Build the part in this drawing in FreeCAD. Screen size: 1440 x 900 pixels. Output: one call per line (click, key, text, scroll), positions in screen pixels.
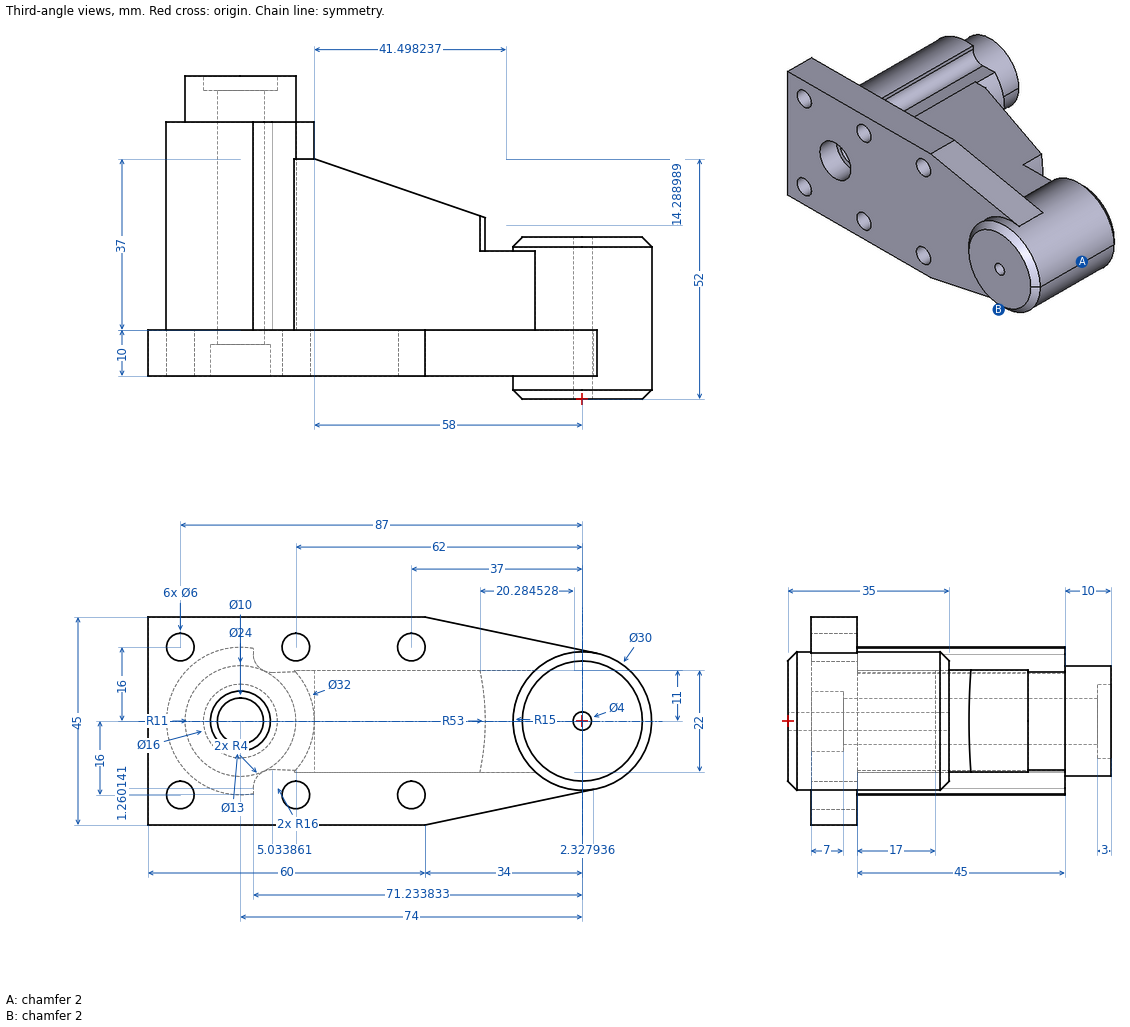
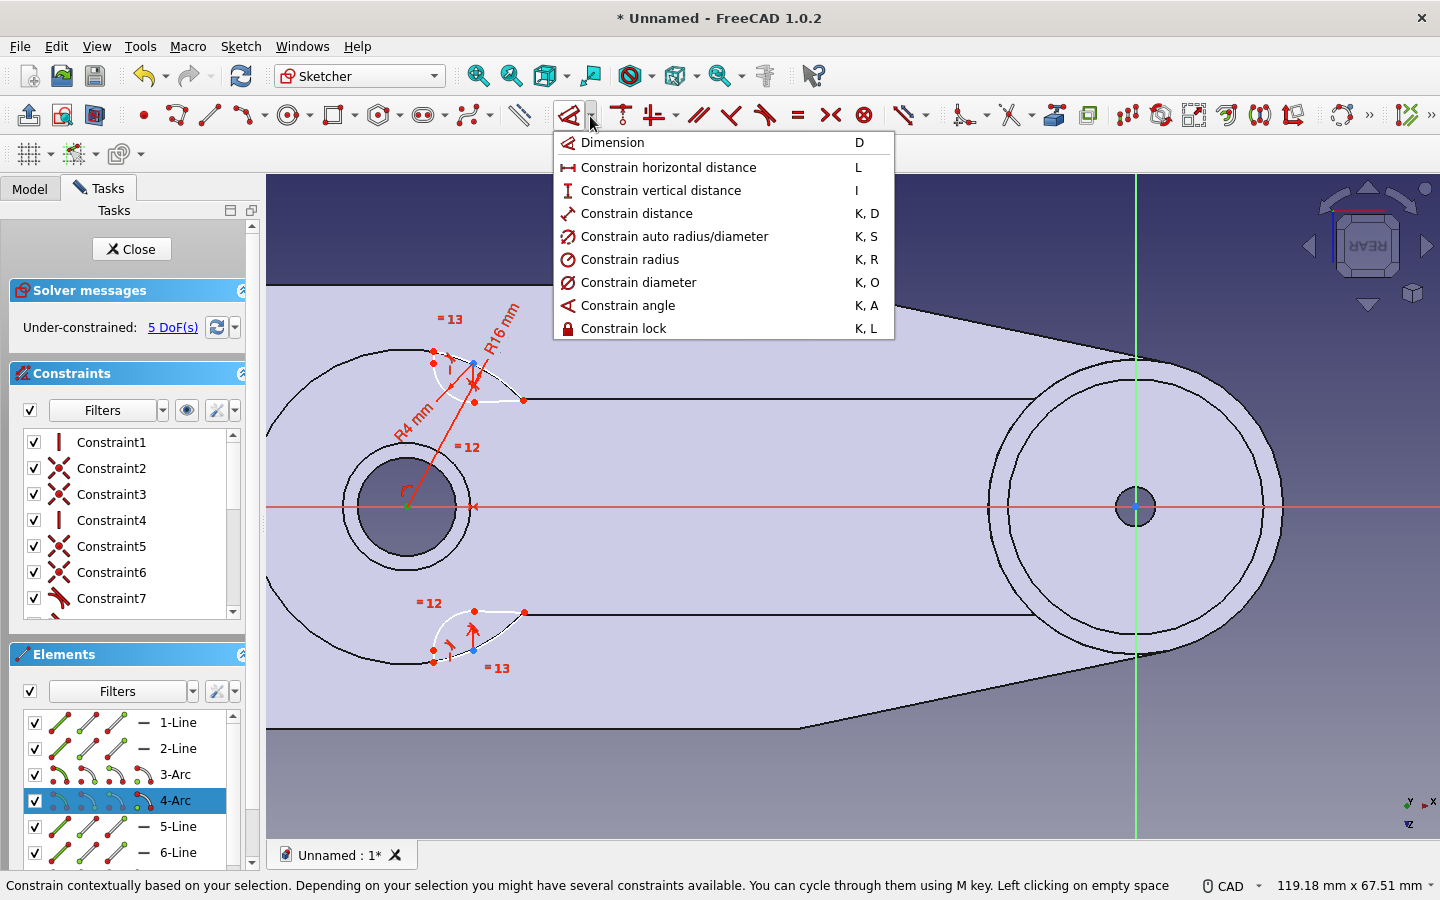
click(724, 168)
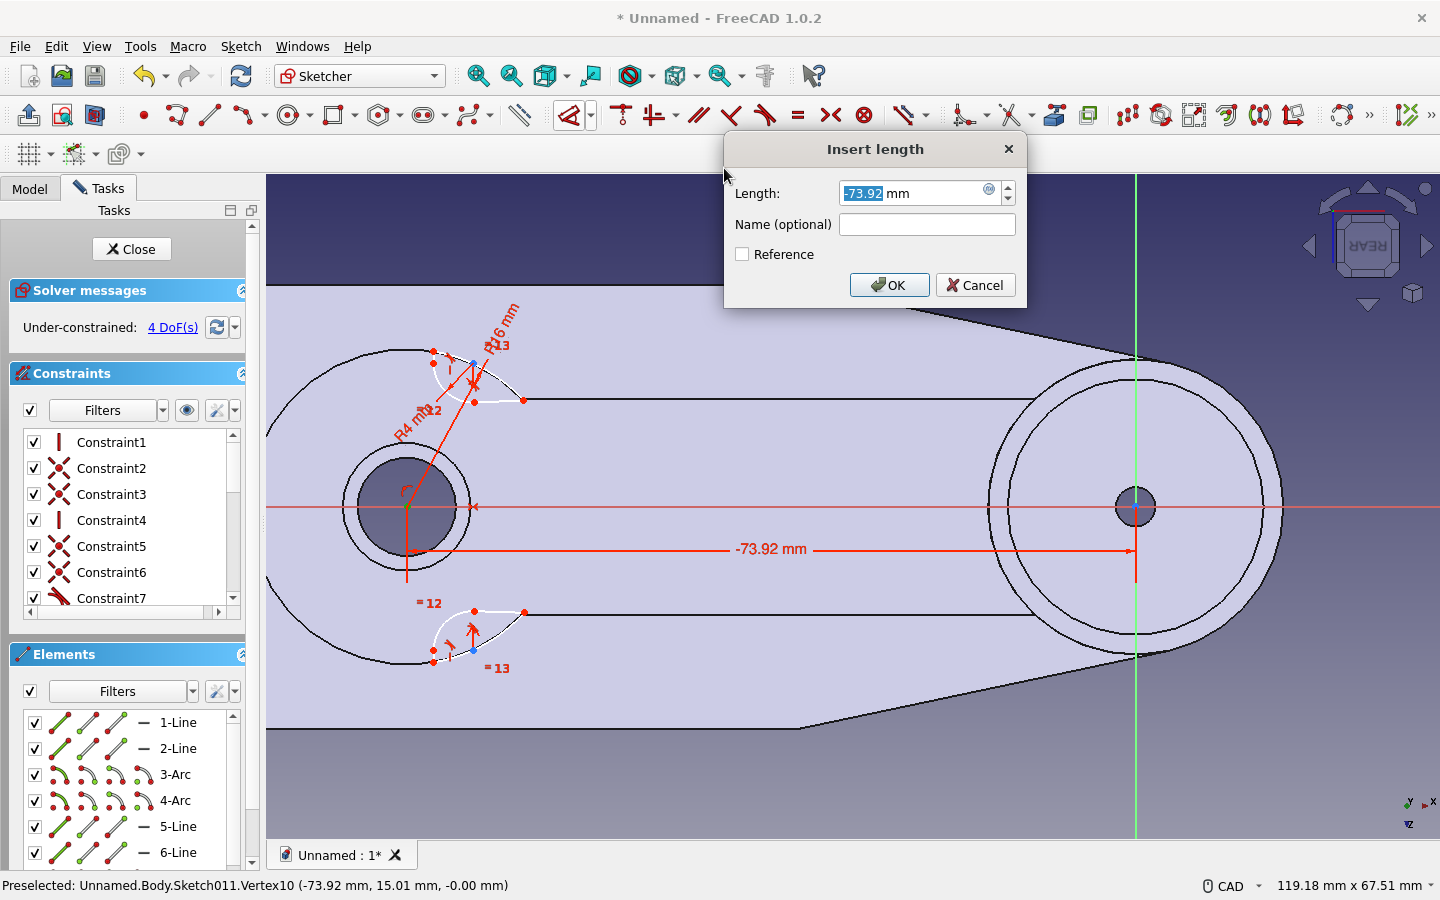
text(-74)
key(Return)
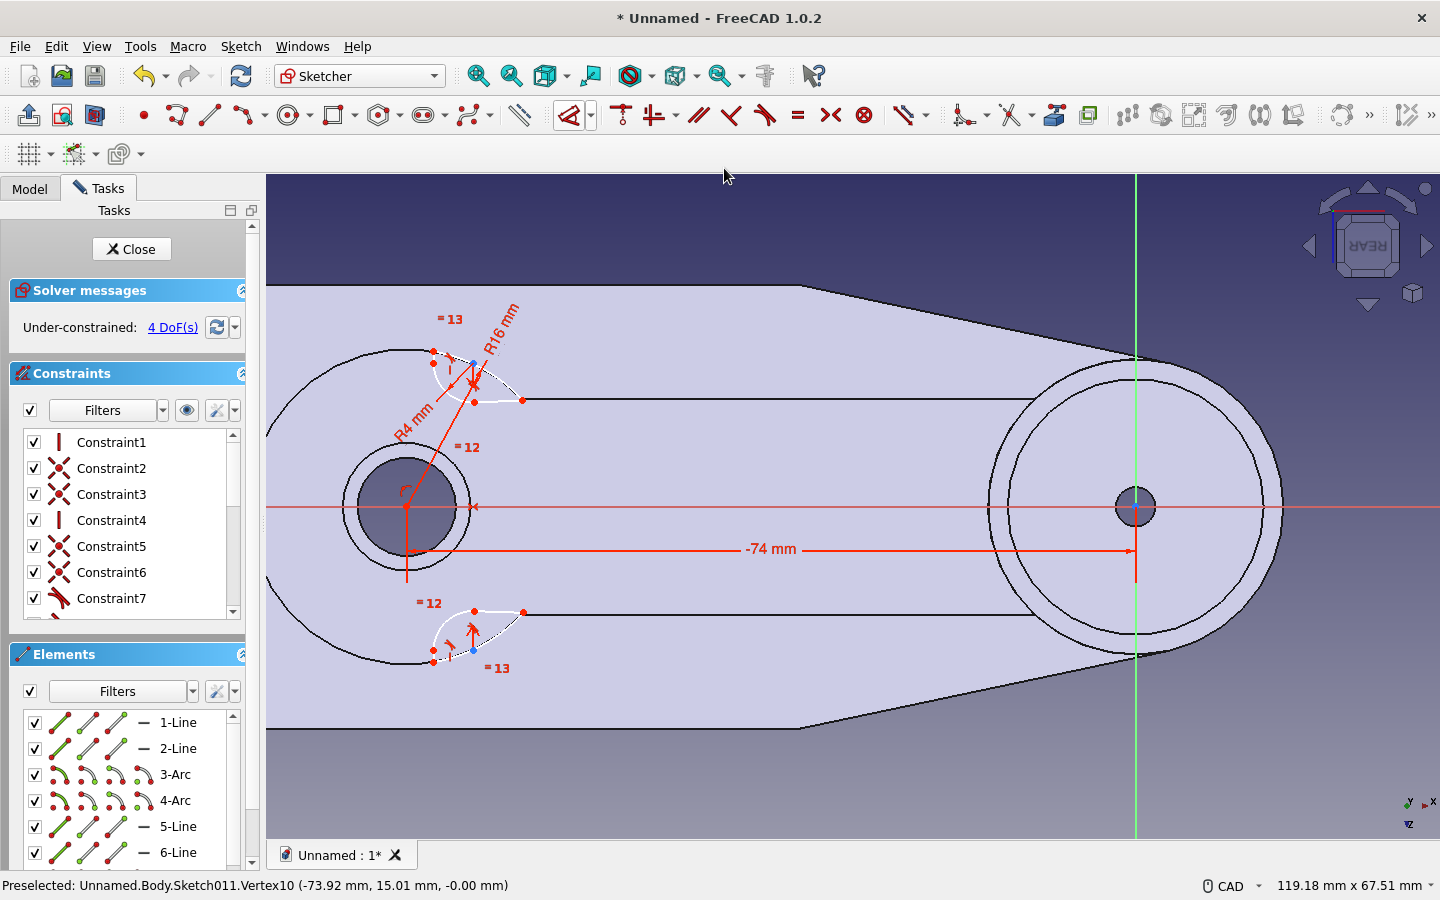
scroll(434, 357, up, 6)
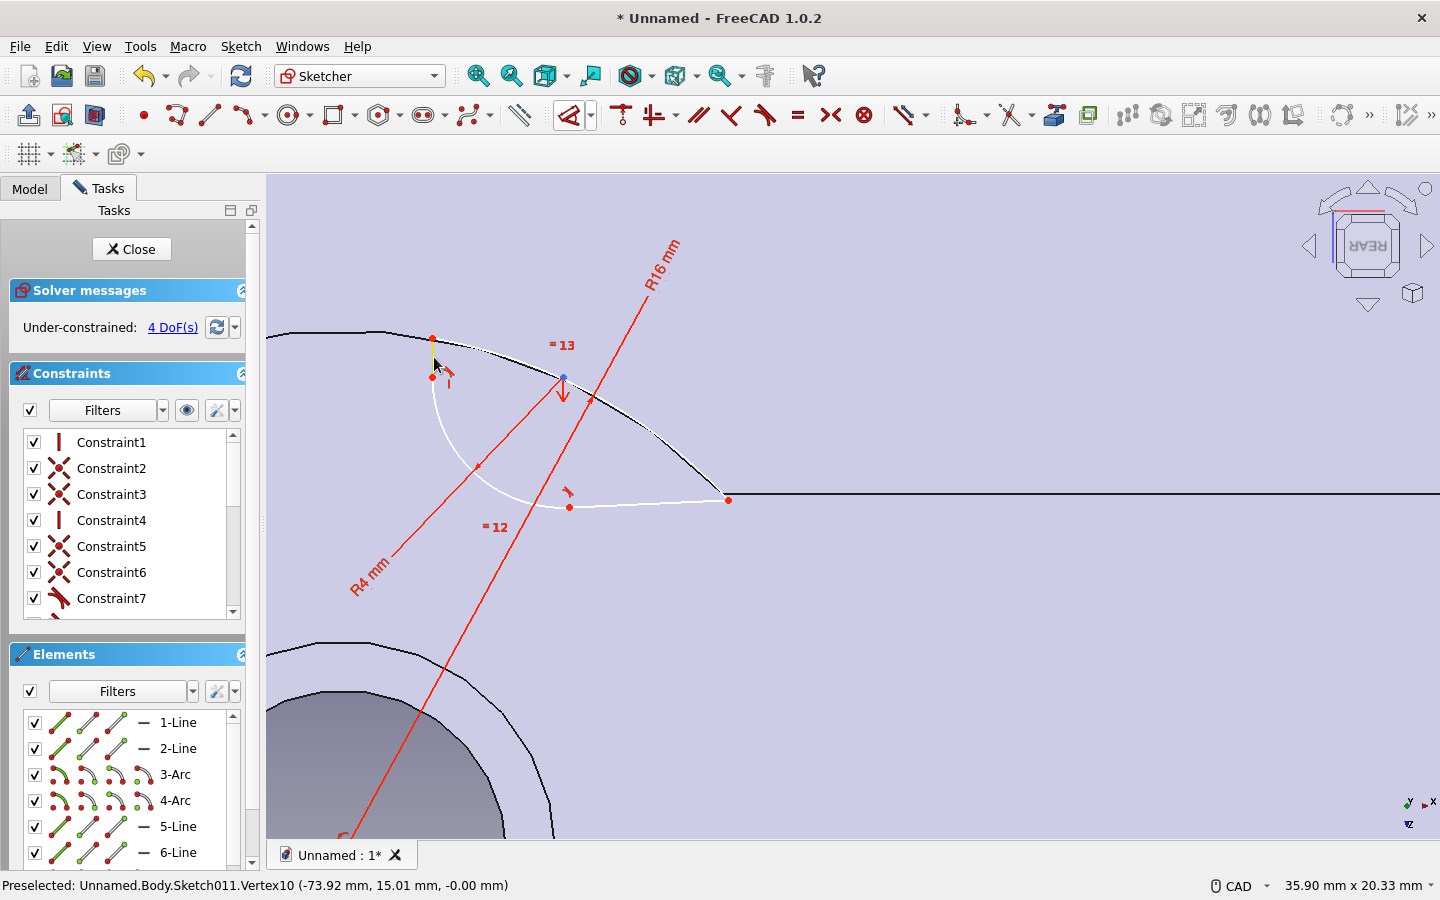
click(433, 358)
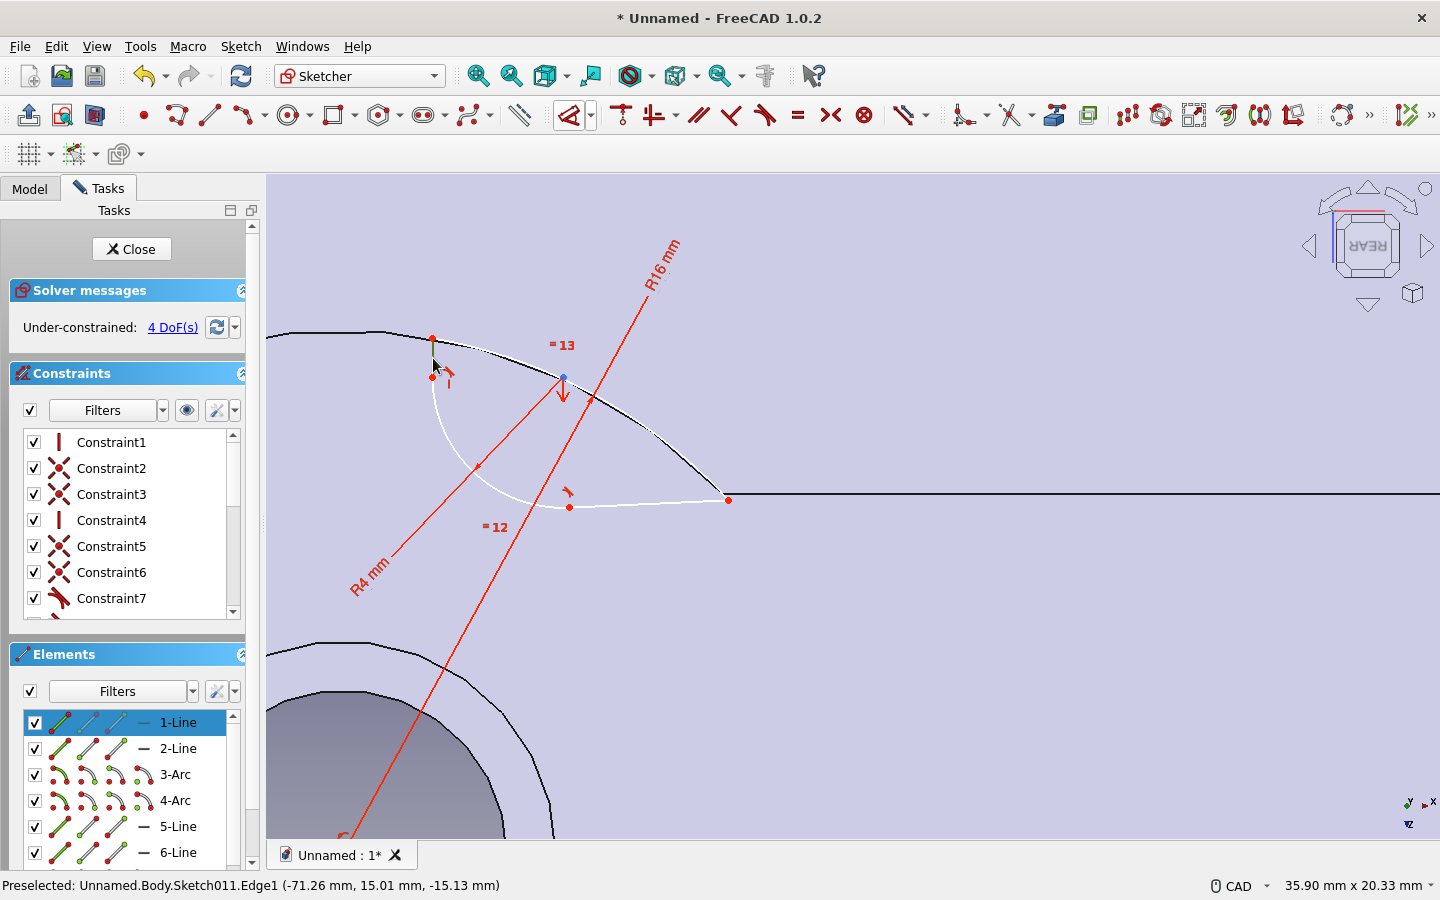
click(590, 116)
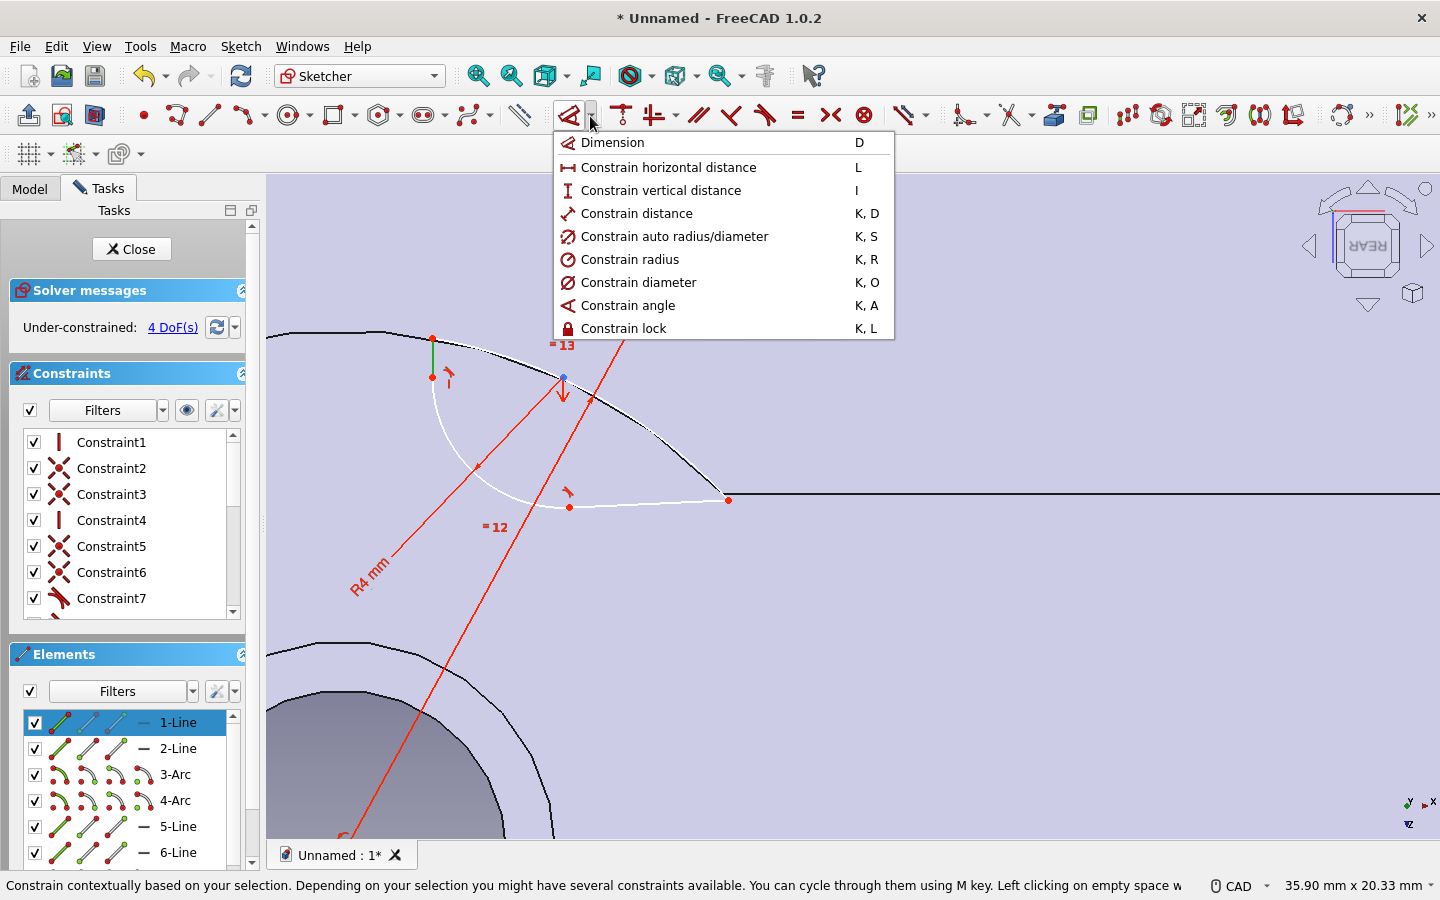
click(724, 190)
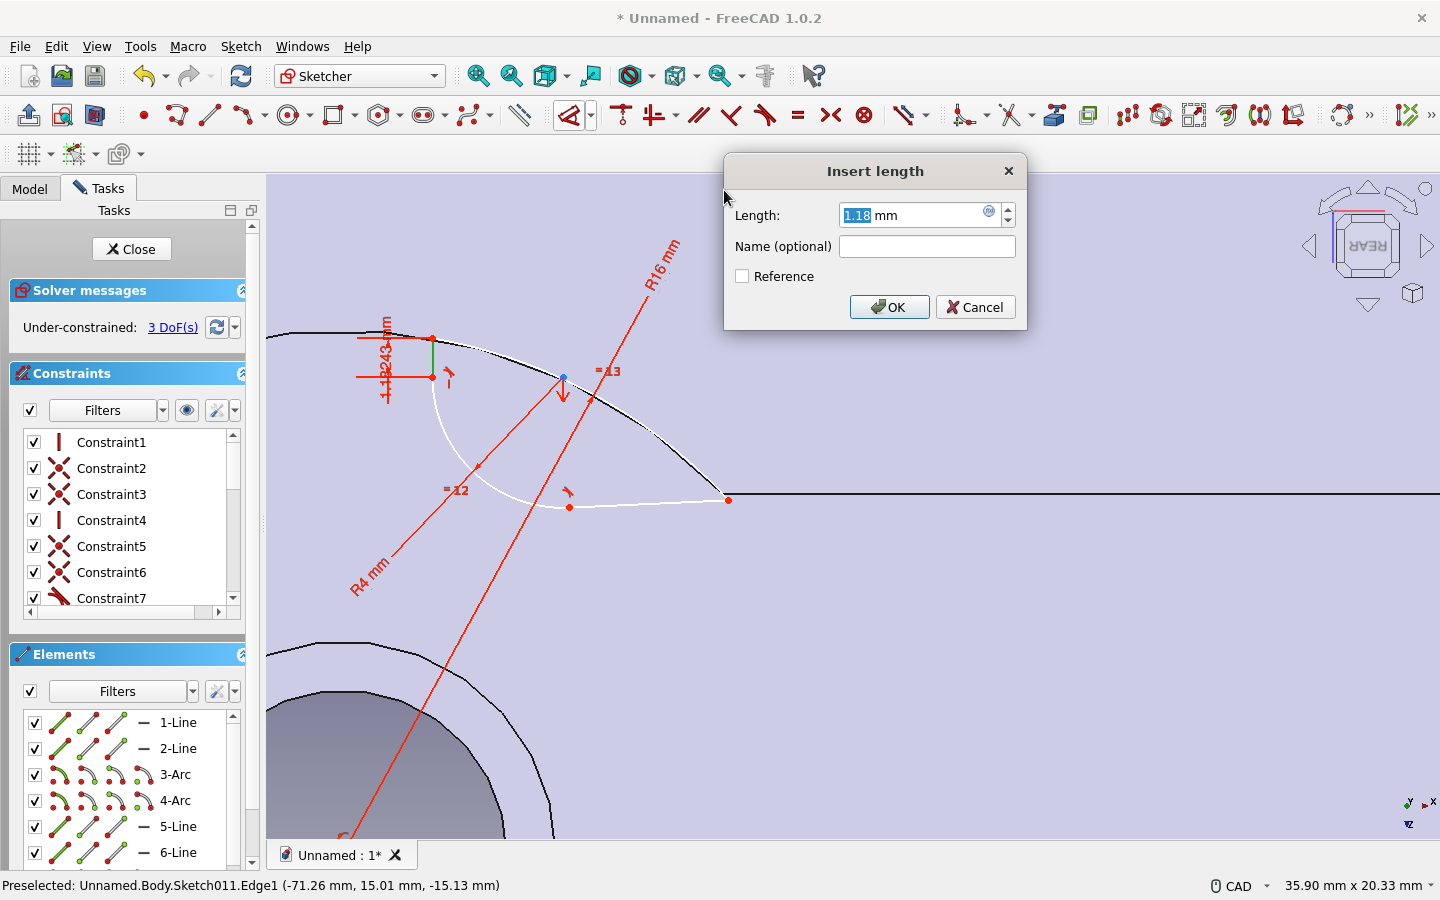
text(1.260141)
key(Return)